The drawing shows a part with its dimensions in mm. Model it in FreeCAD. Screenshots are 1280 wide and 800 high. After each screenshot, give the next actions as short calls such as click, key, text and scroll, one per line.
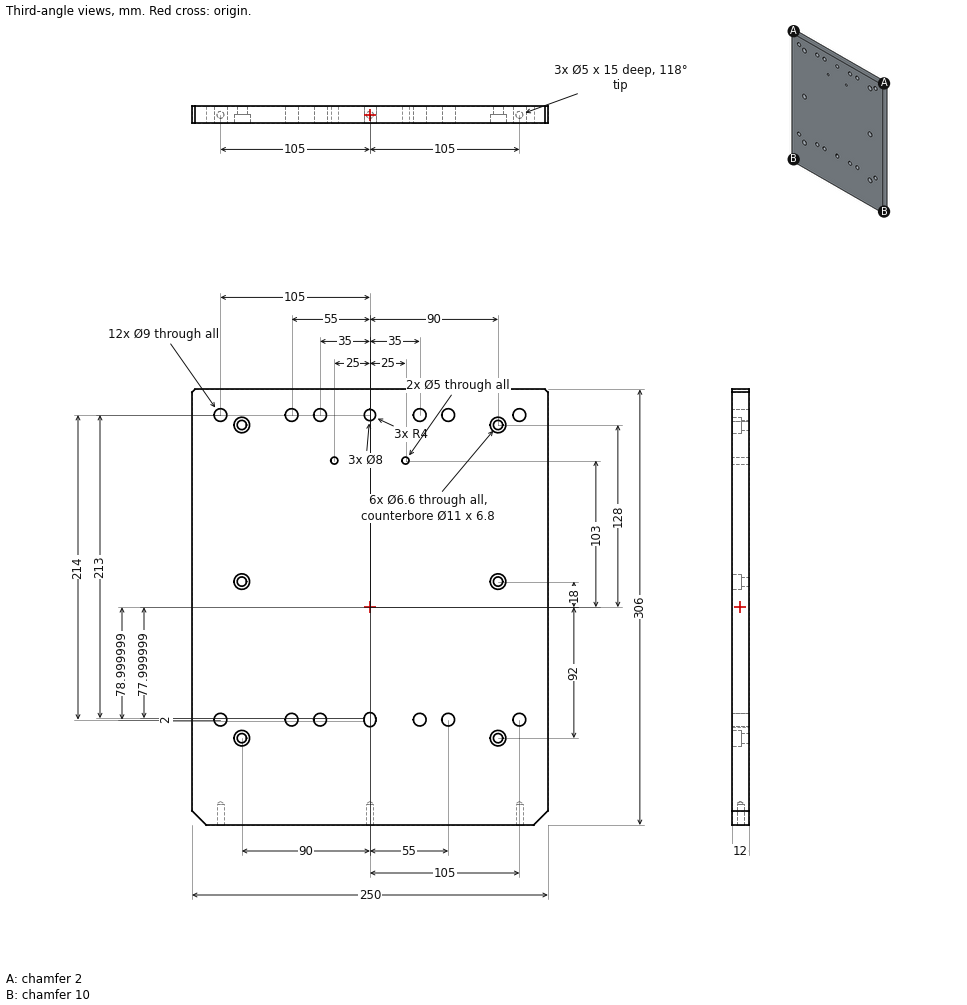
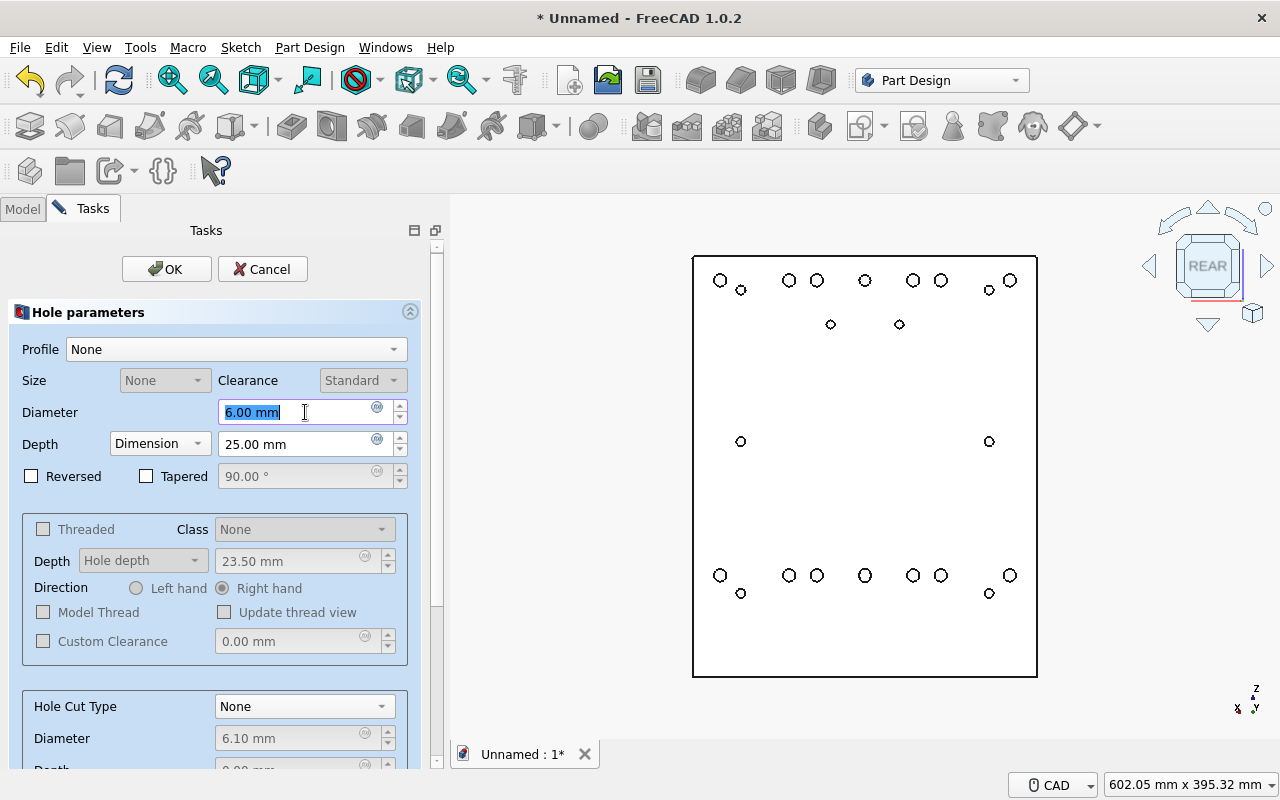
text(5)
key(Tab)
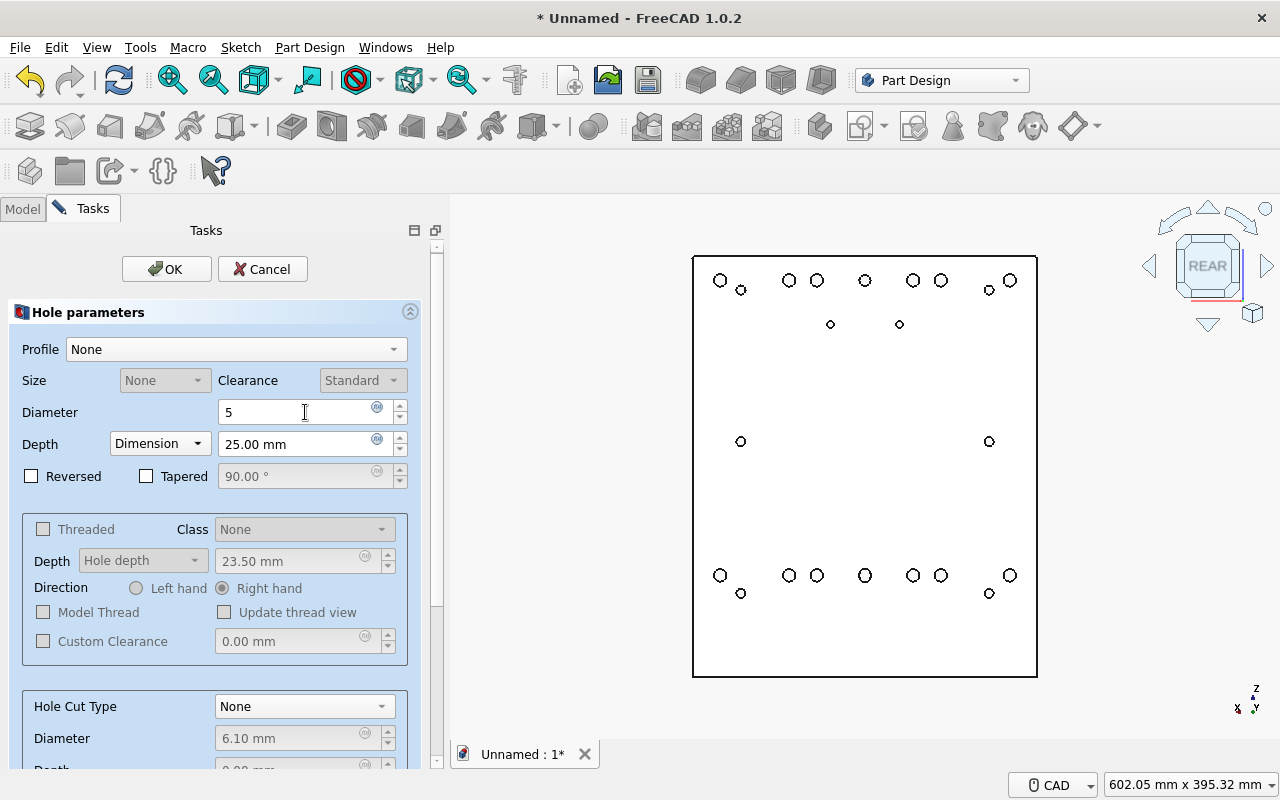
click(161, 444)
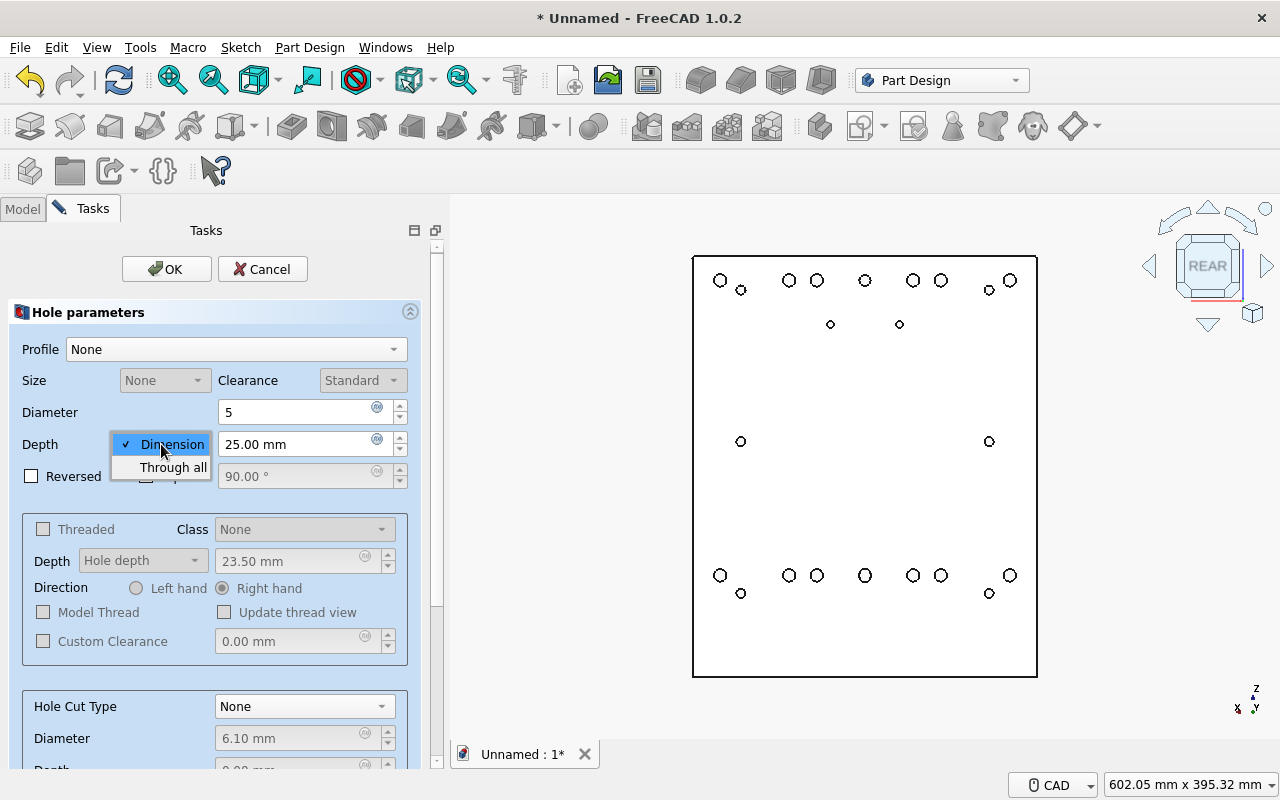
click(160, 468)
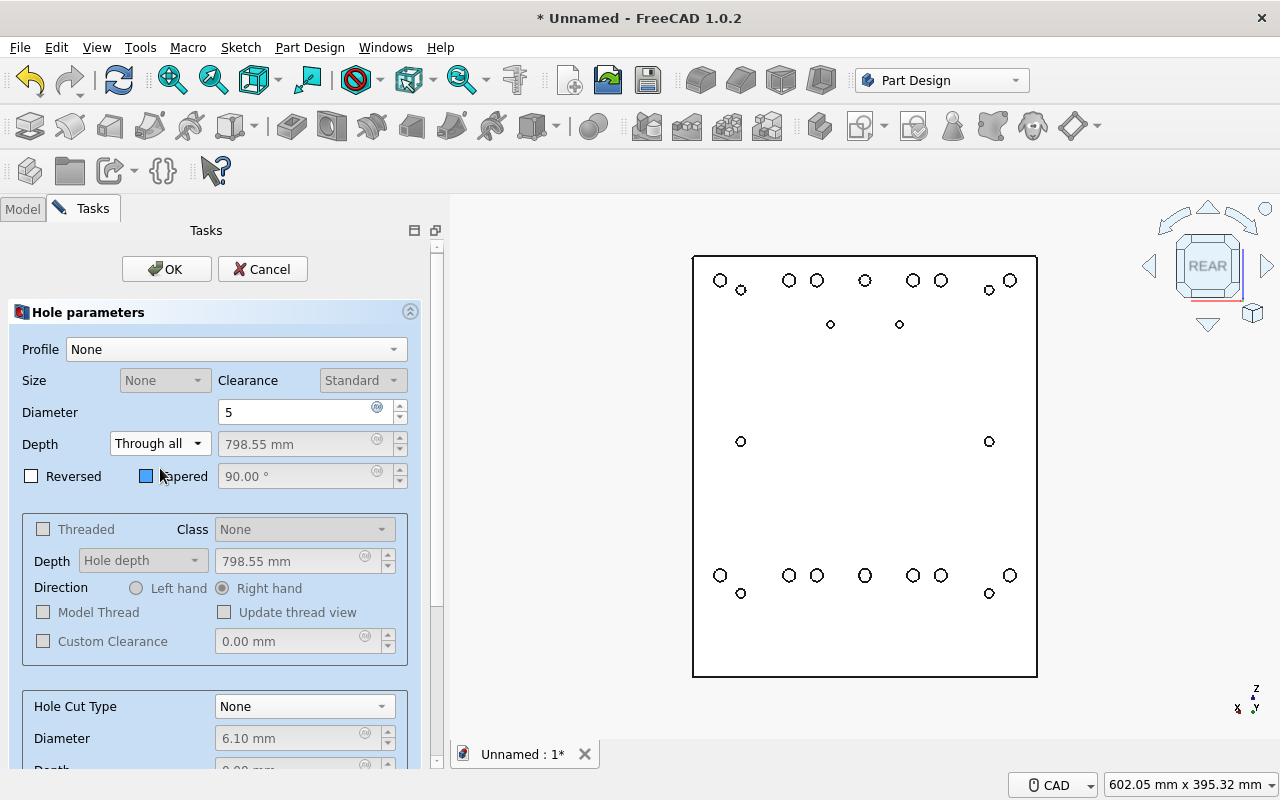
click(167, 269)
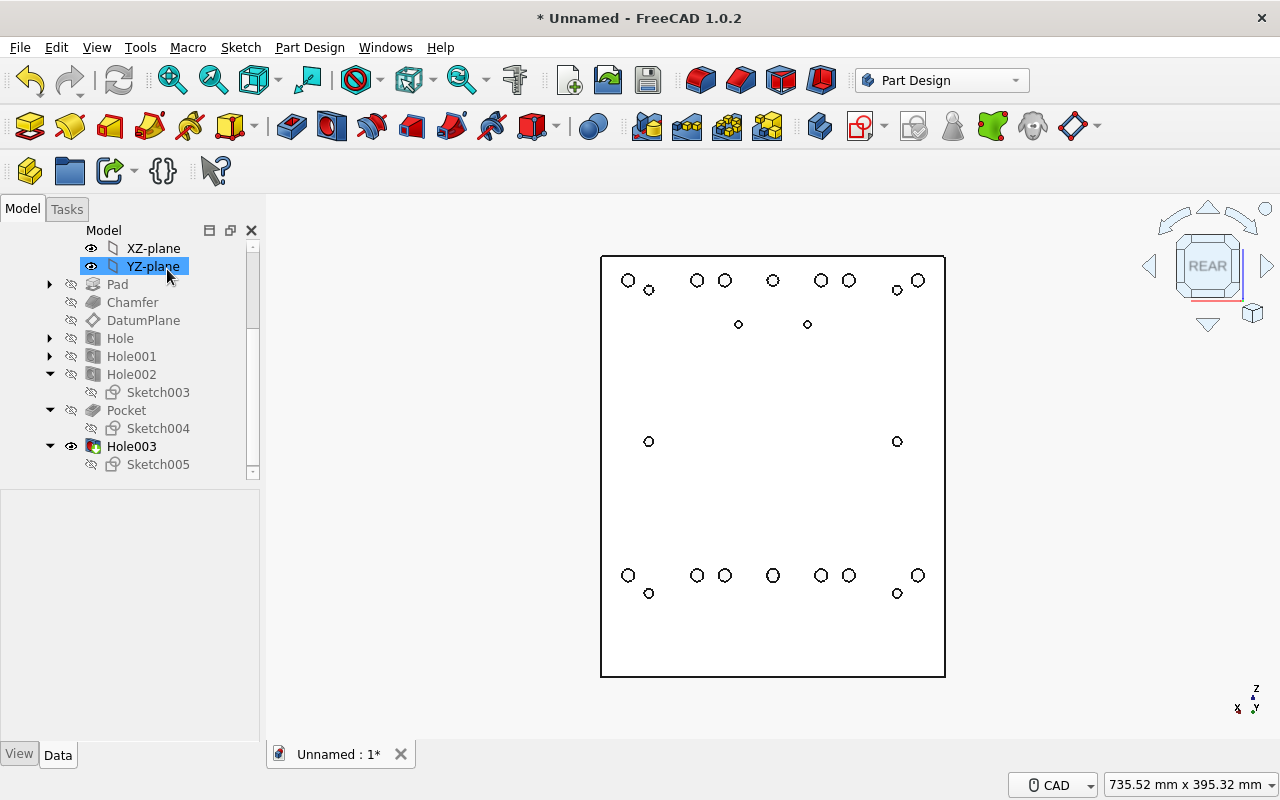
scroll(945, 676, up, 5)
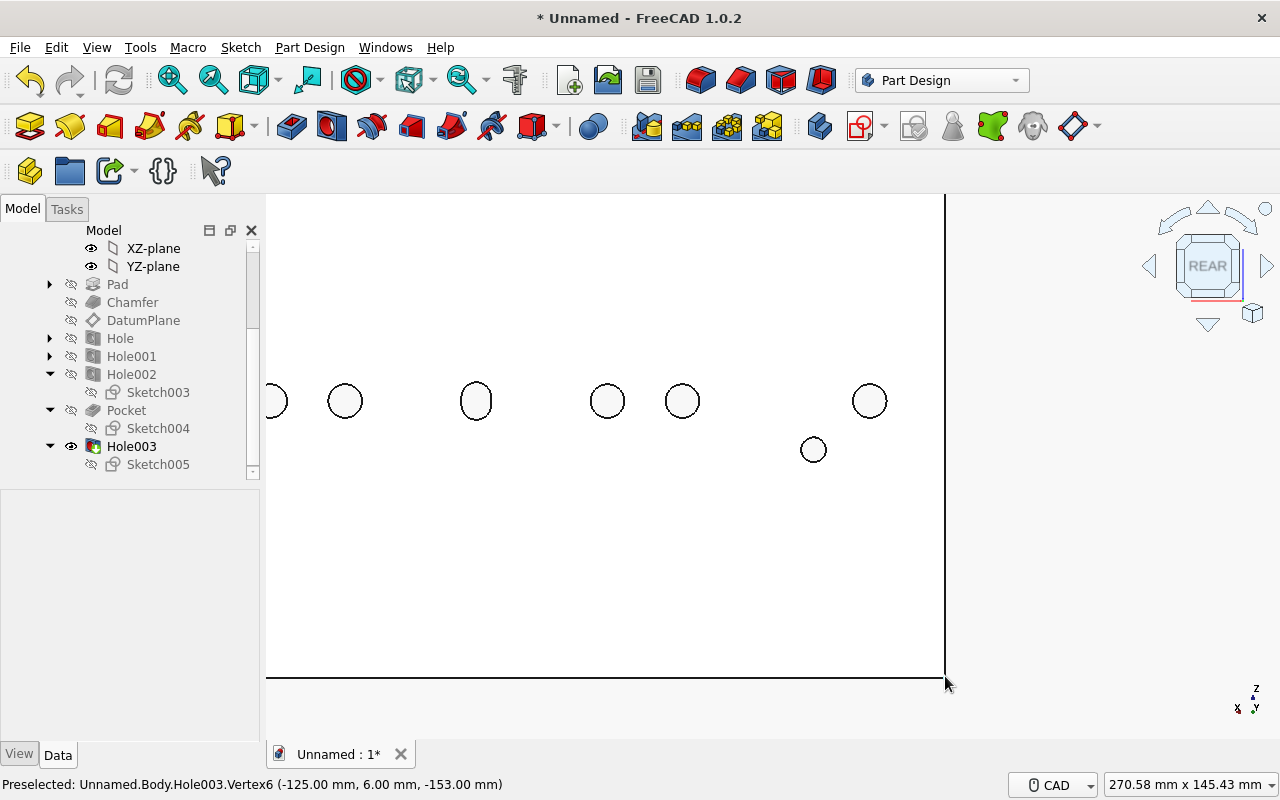
key(v)
key(f)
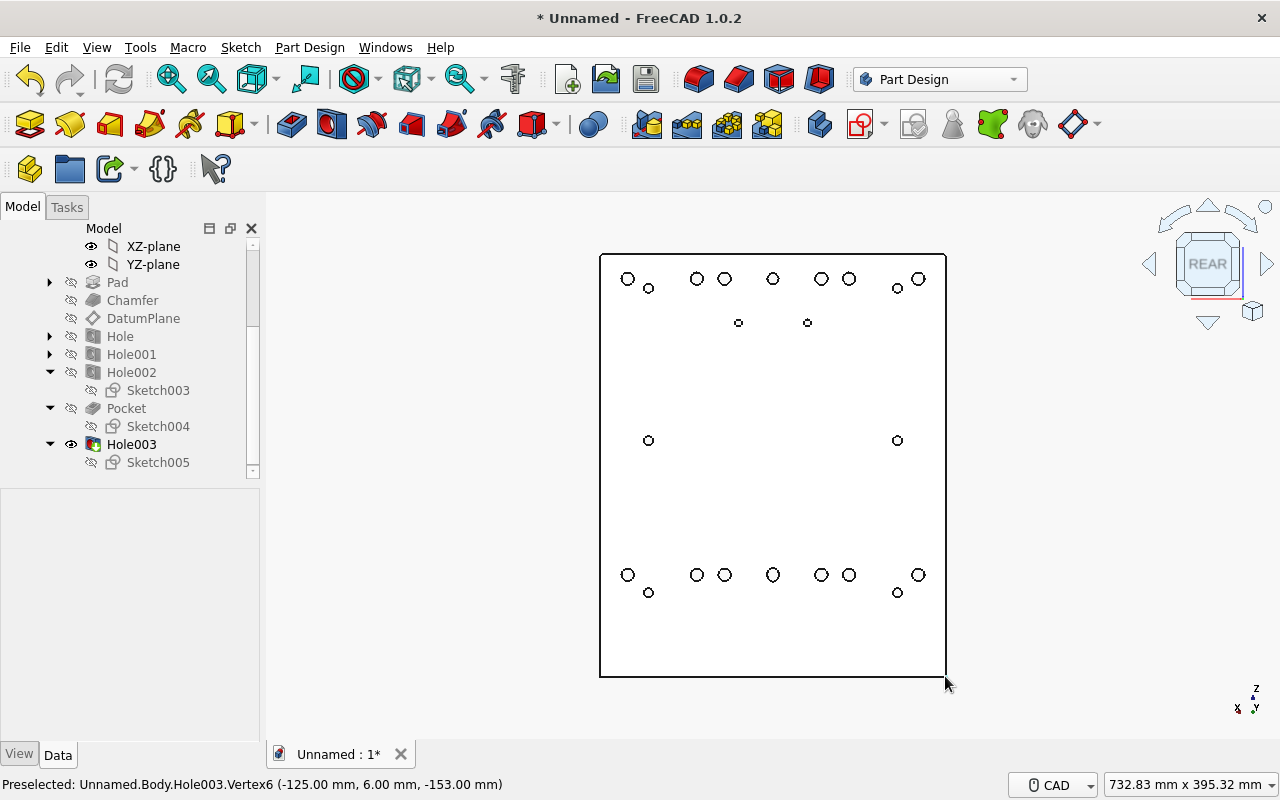
key(0)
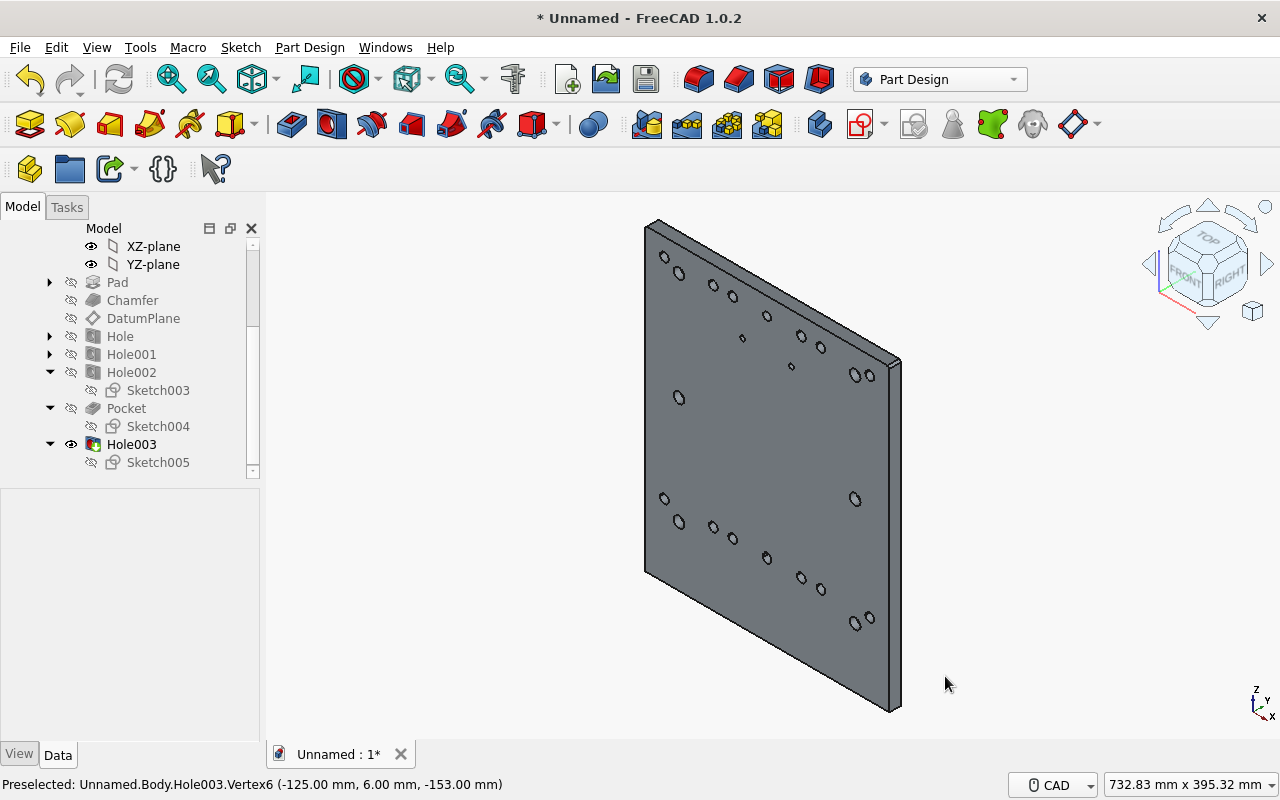
scroll(651, 567, up, 5)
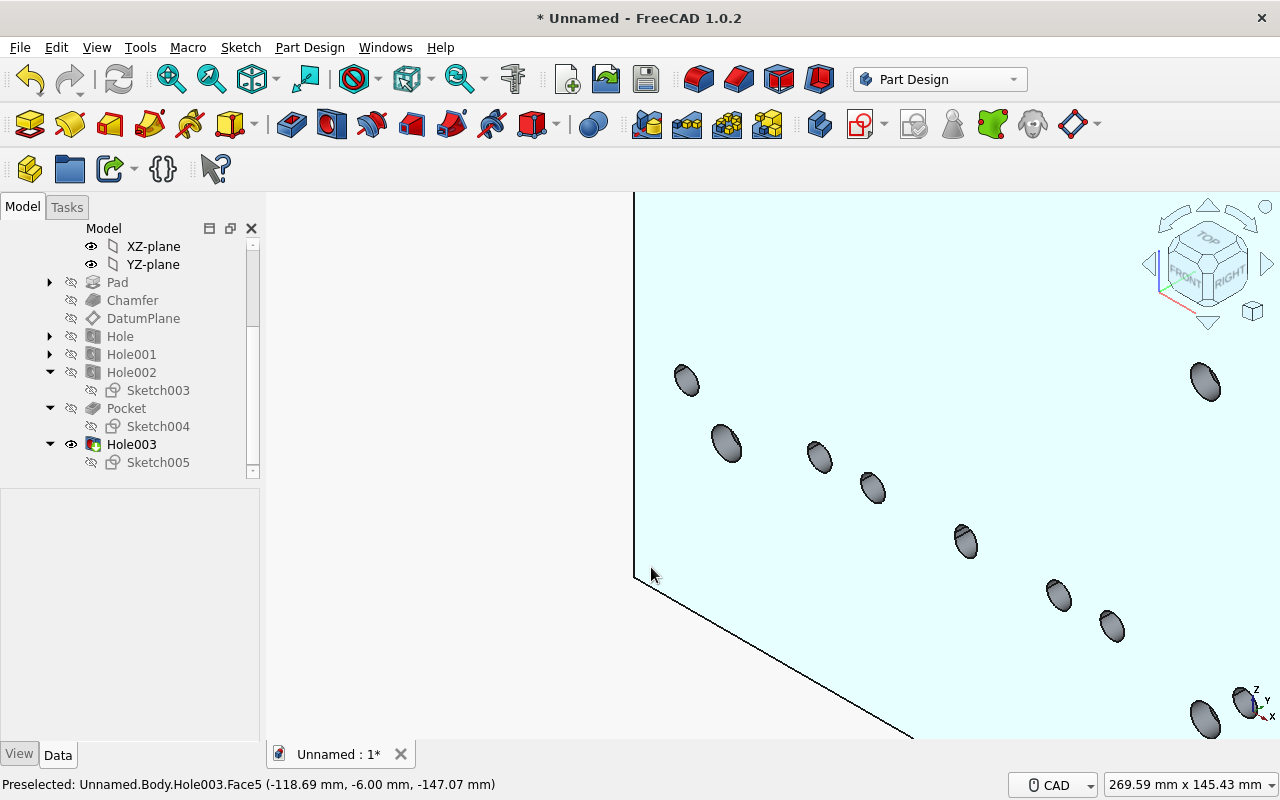
click(172, 80)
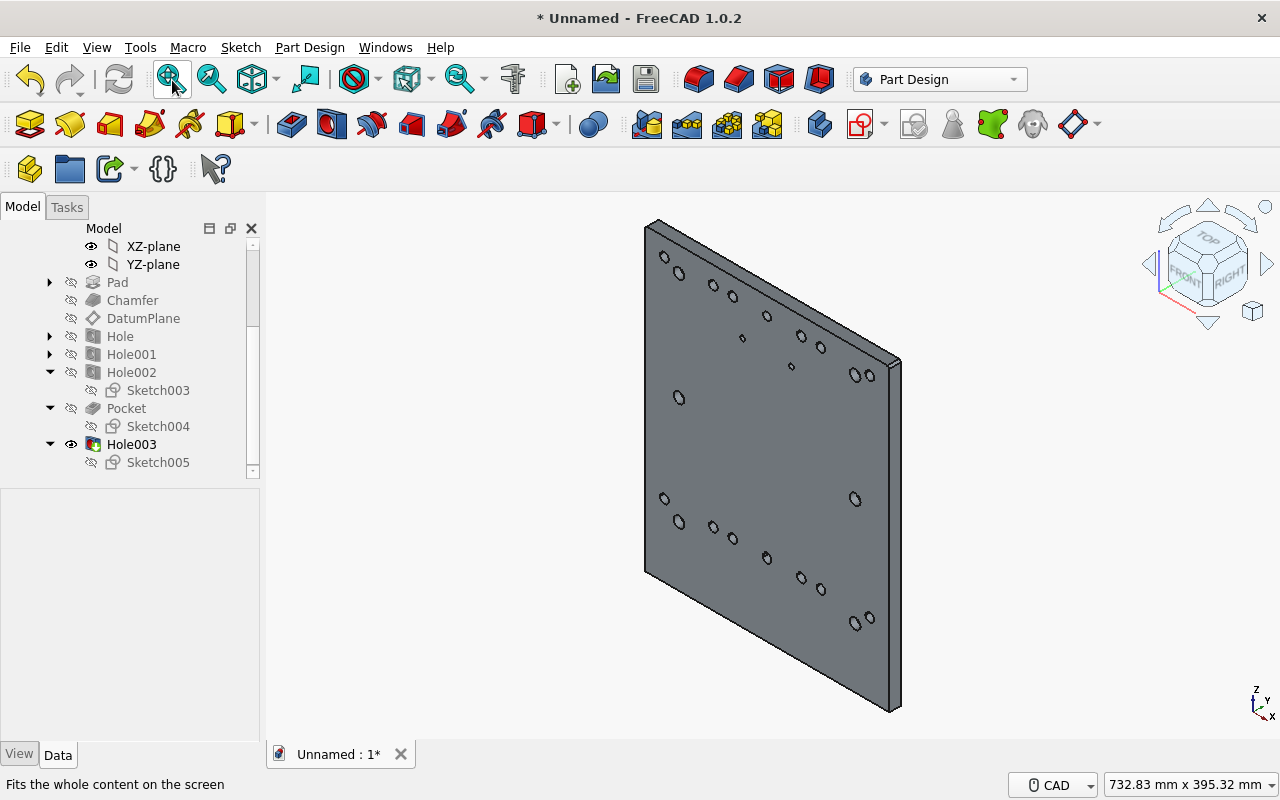
key(2)